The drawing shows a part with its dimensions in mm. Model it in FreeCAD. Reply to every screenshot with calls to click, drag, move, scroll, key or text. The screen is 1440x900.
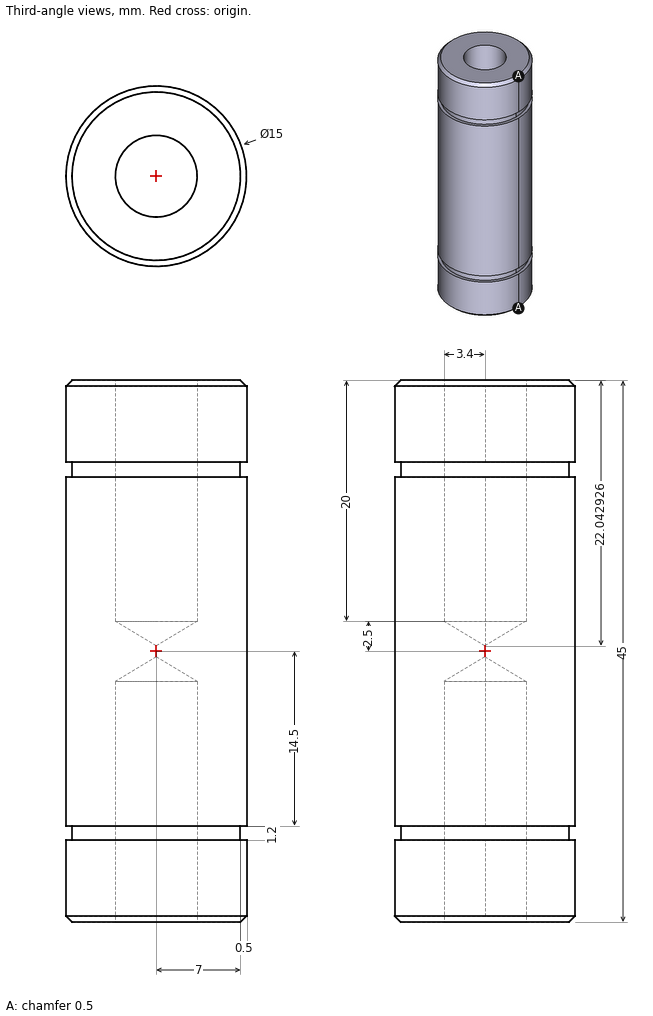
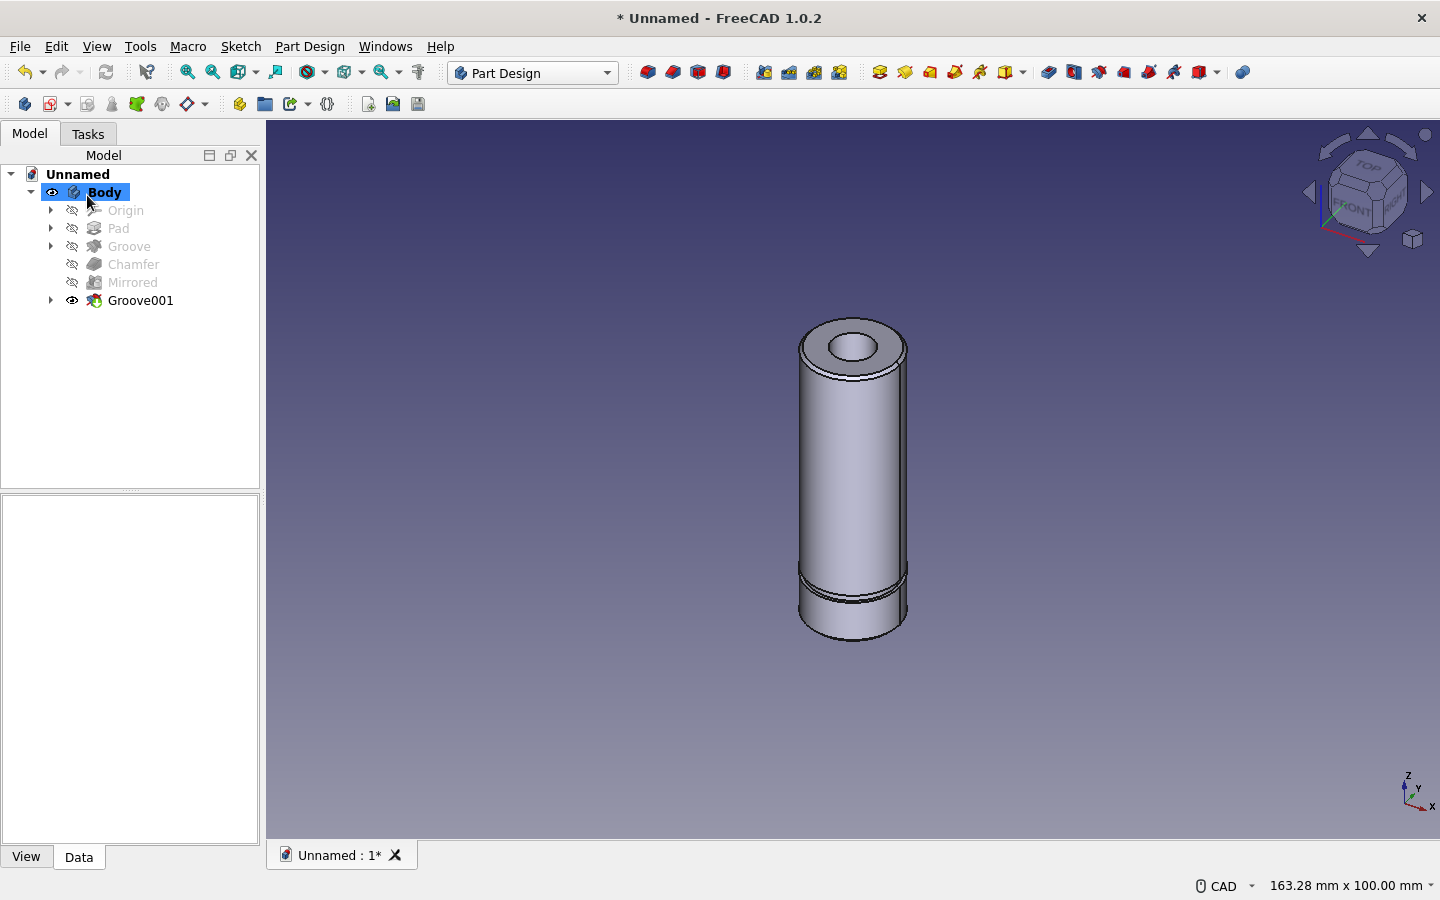
click(117, 300)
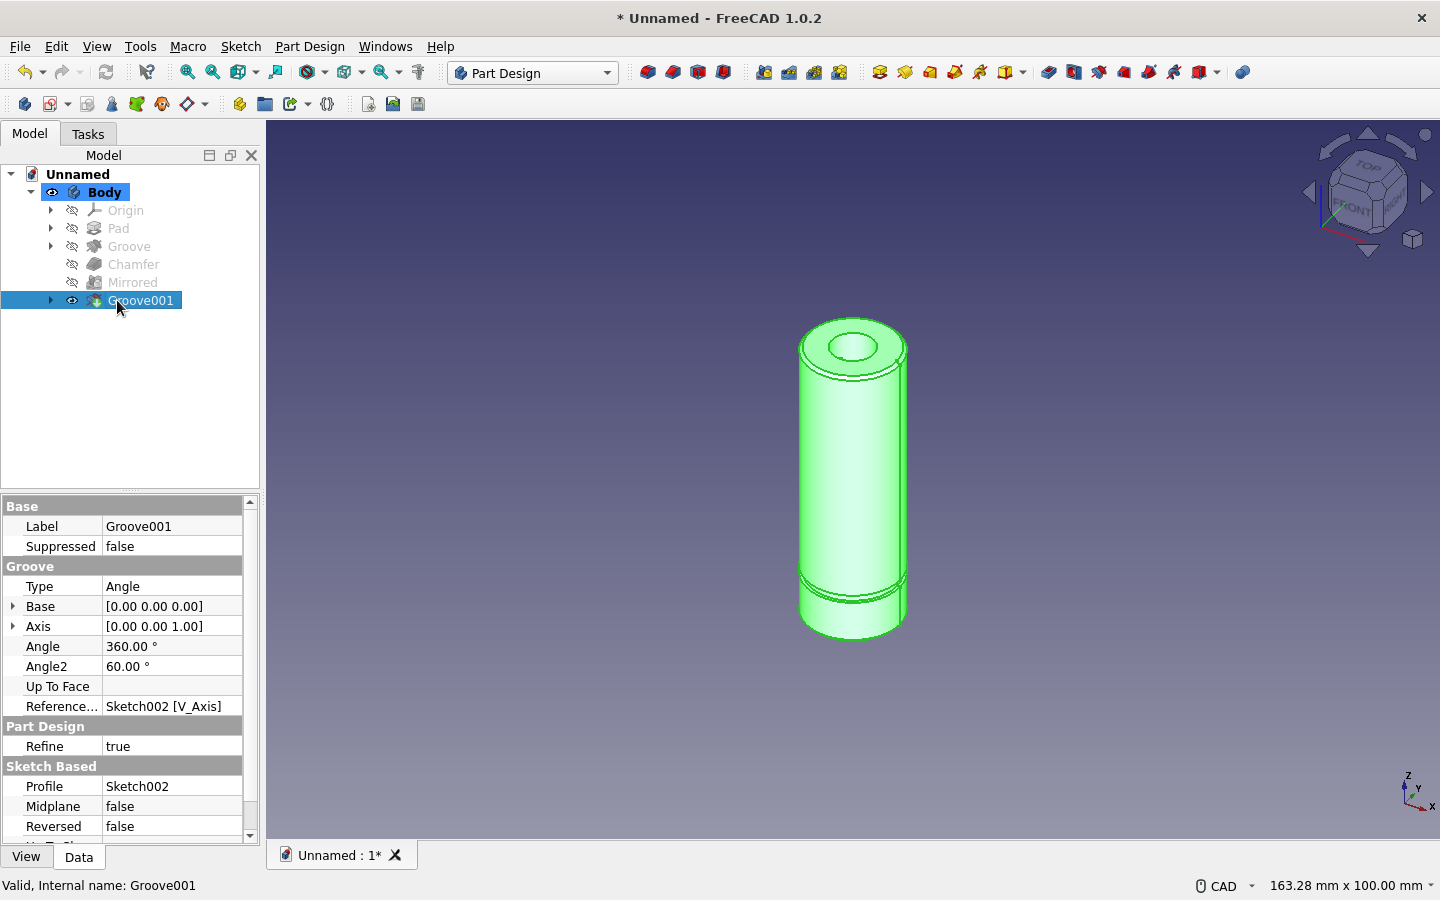
click(764, 72)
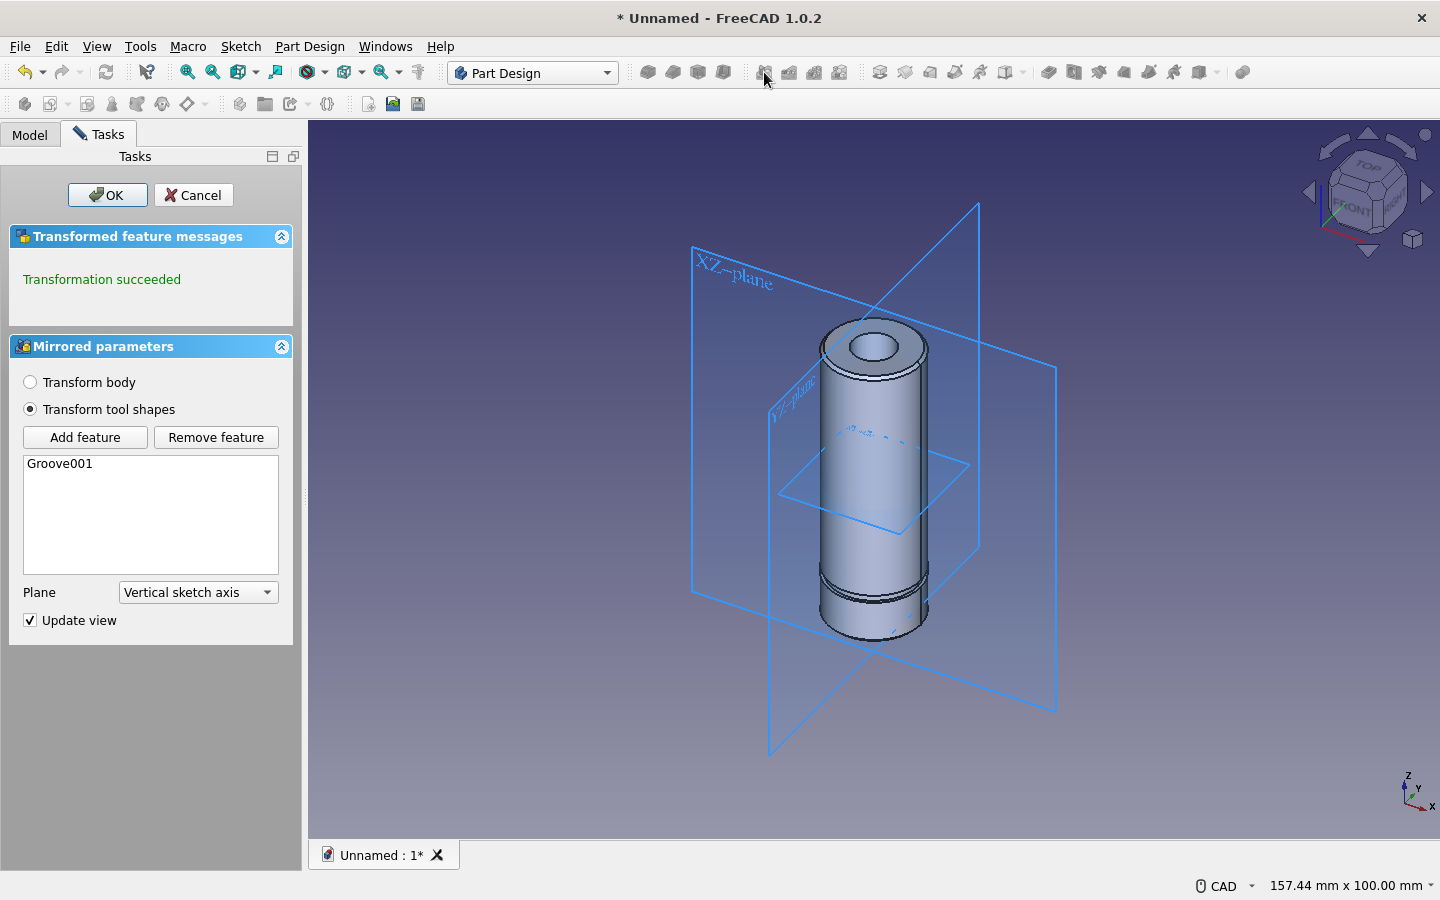
click(199, 592)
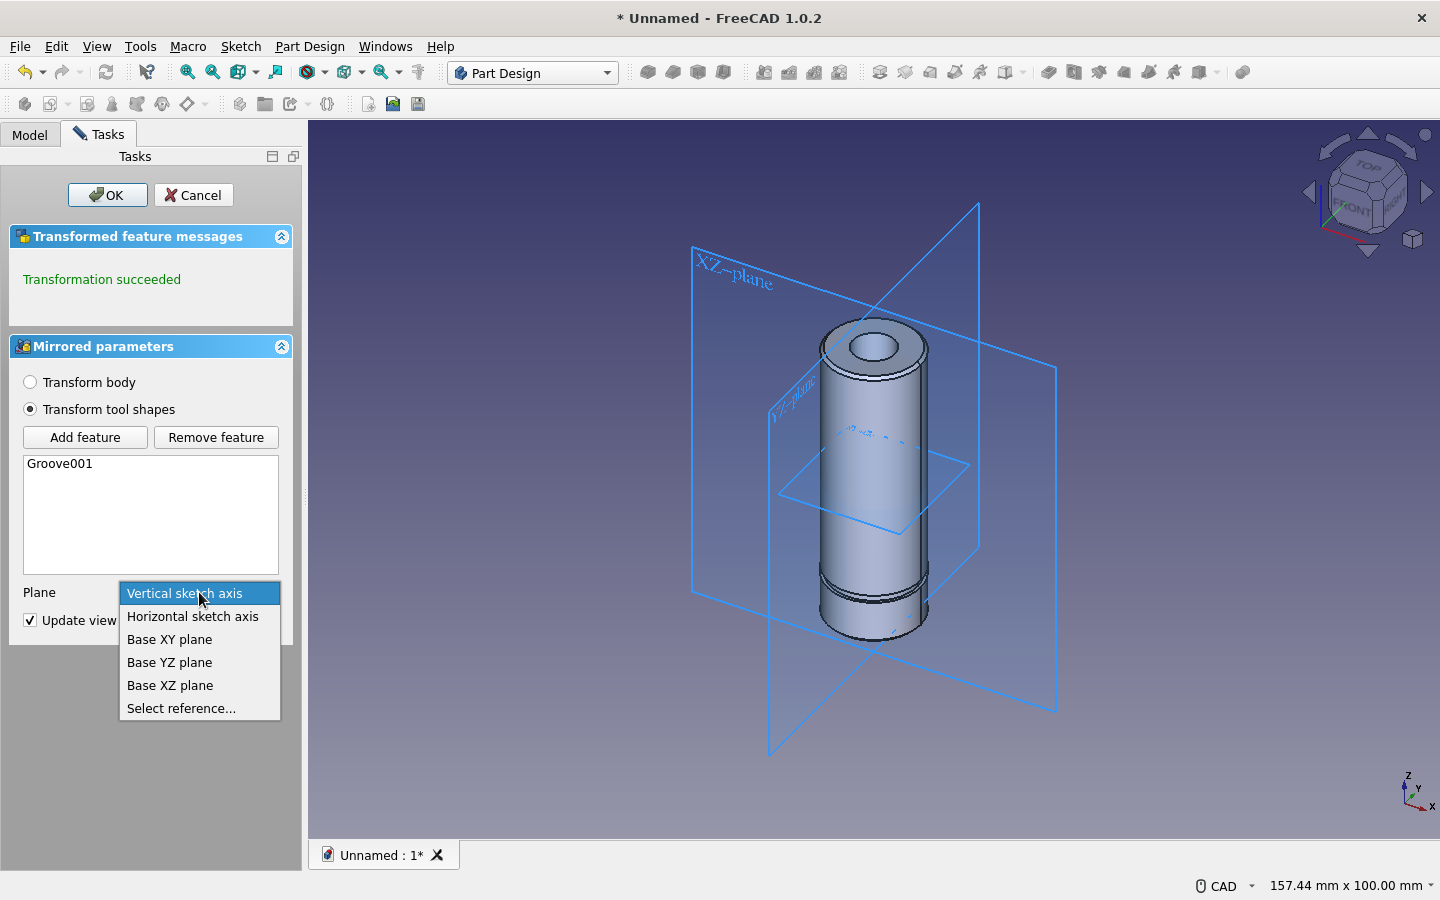
click(198, 640)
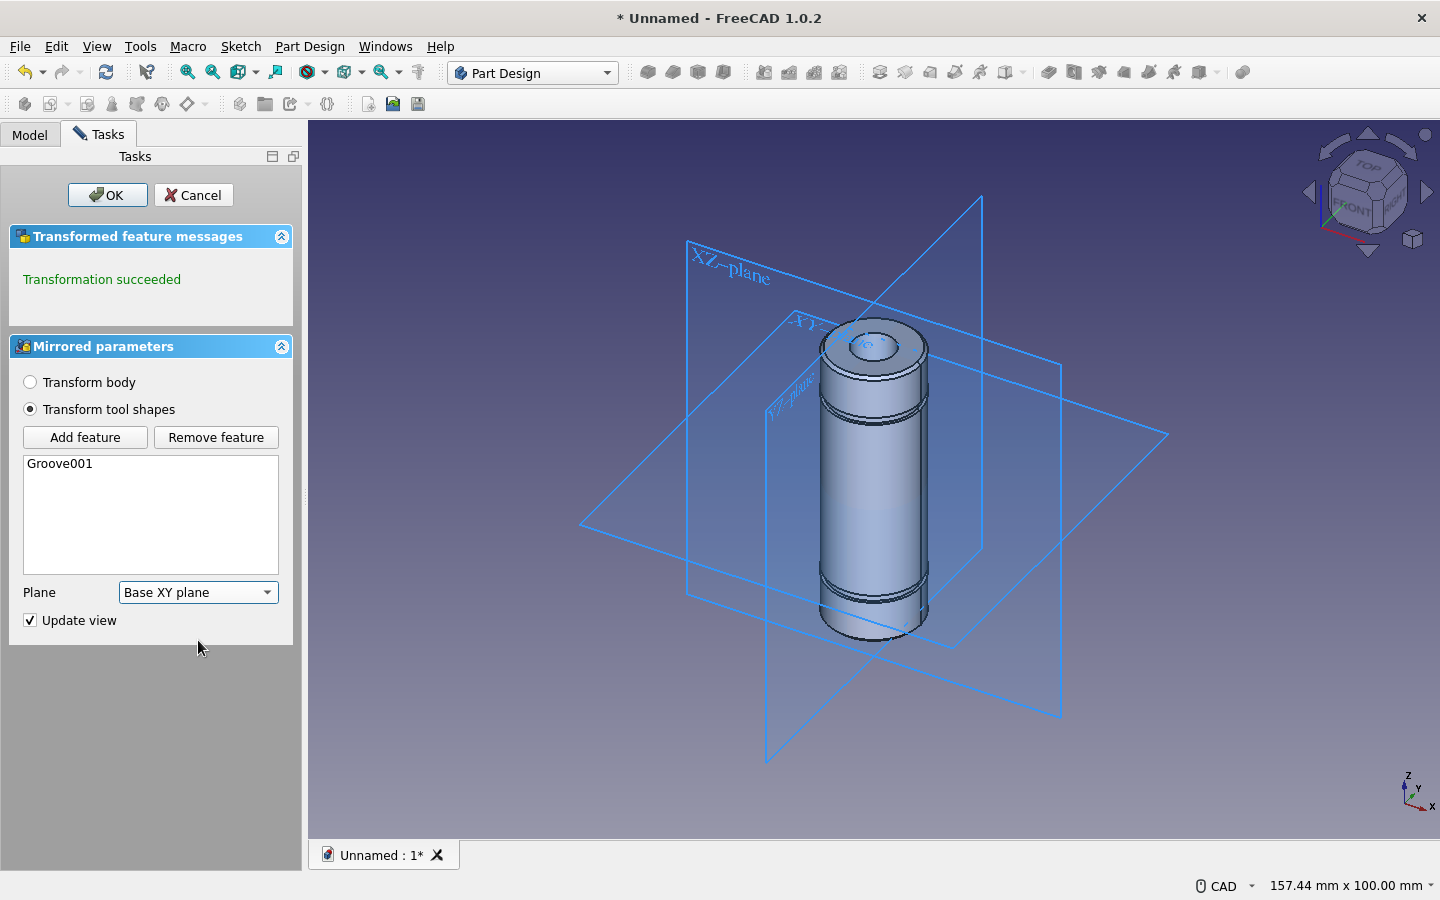
click(108, 195)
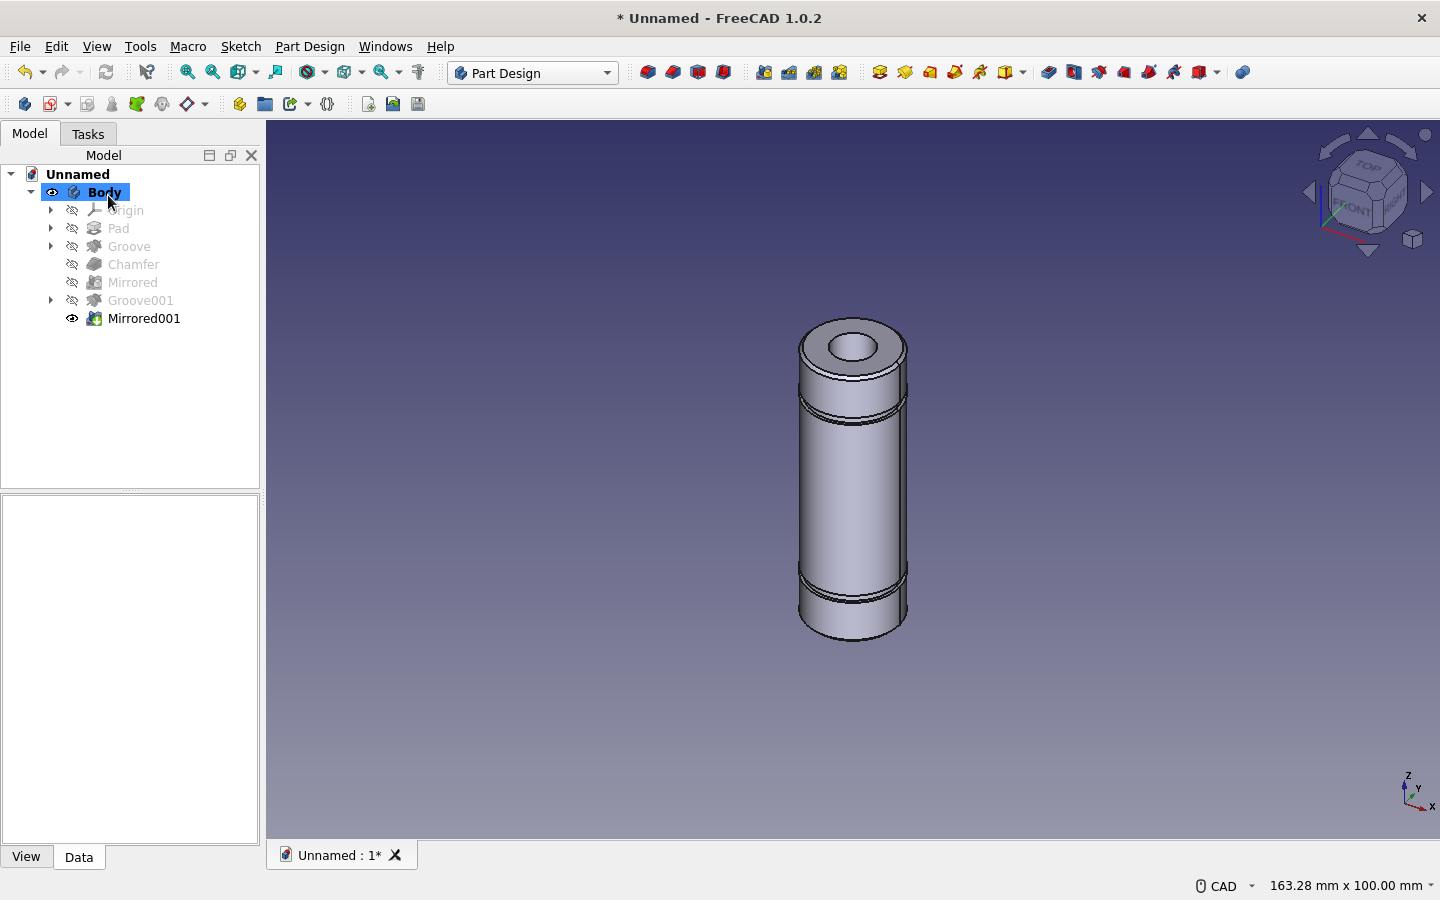
key(0)